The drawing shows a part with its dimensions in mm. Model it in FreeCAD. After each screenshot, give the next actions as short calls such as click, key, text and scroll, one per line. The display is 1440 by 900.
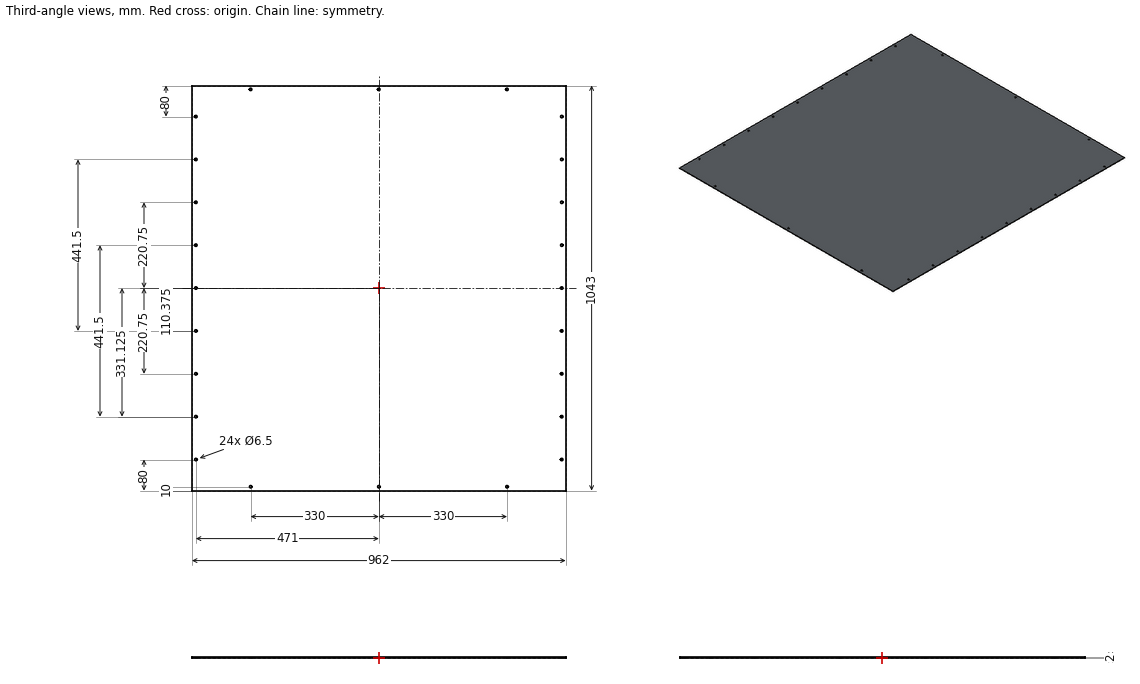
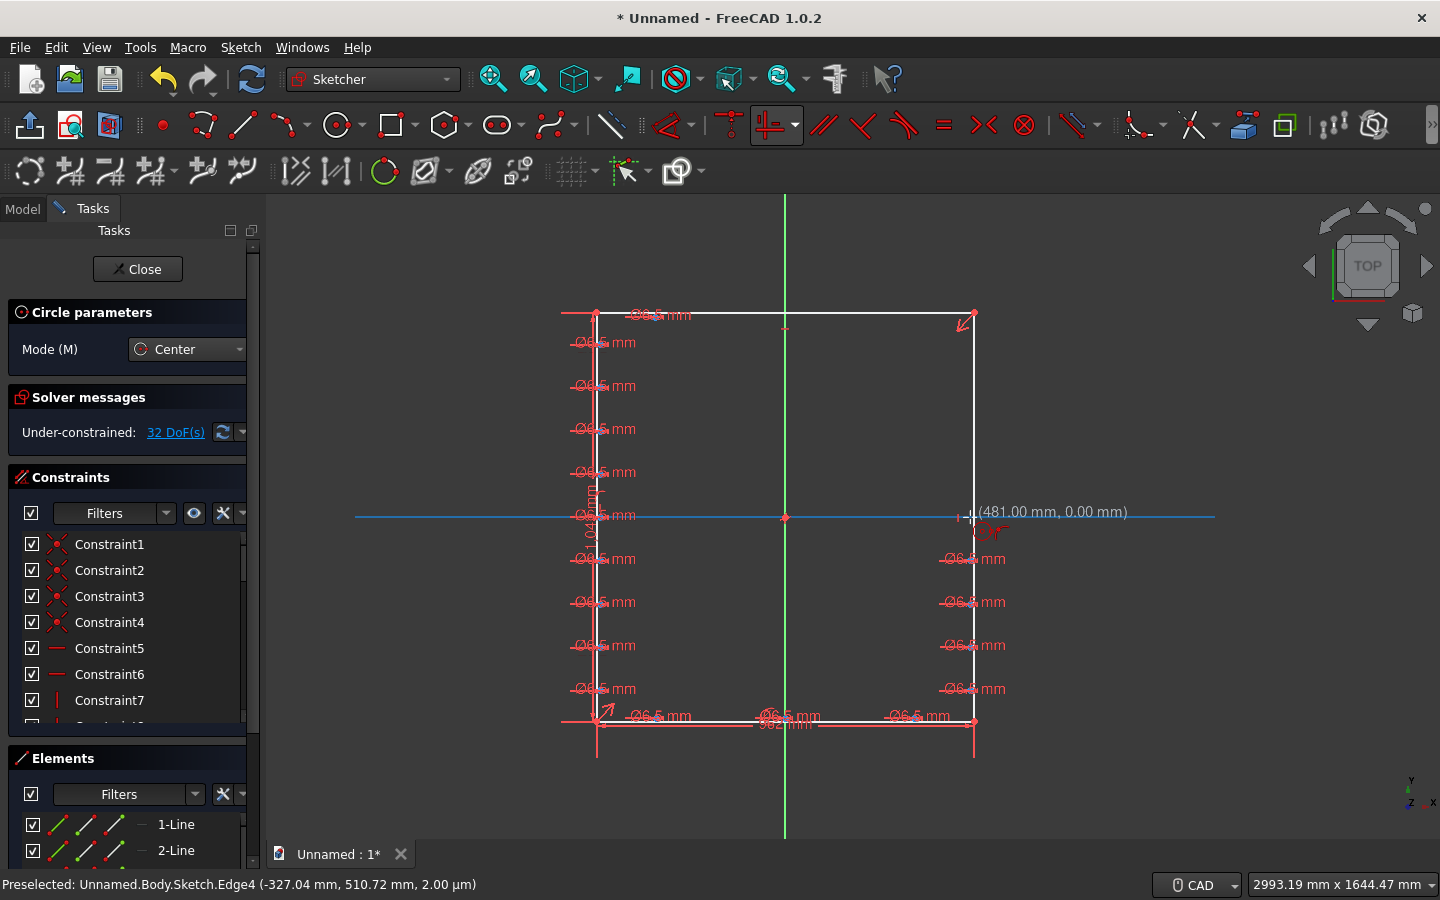
scroll(970, 517, up, 7)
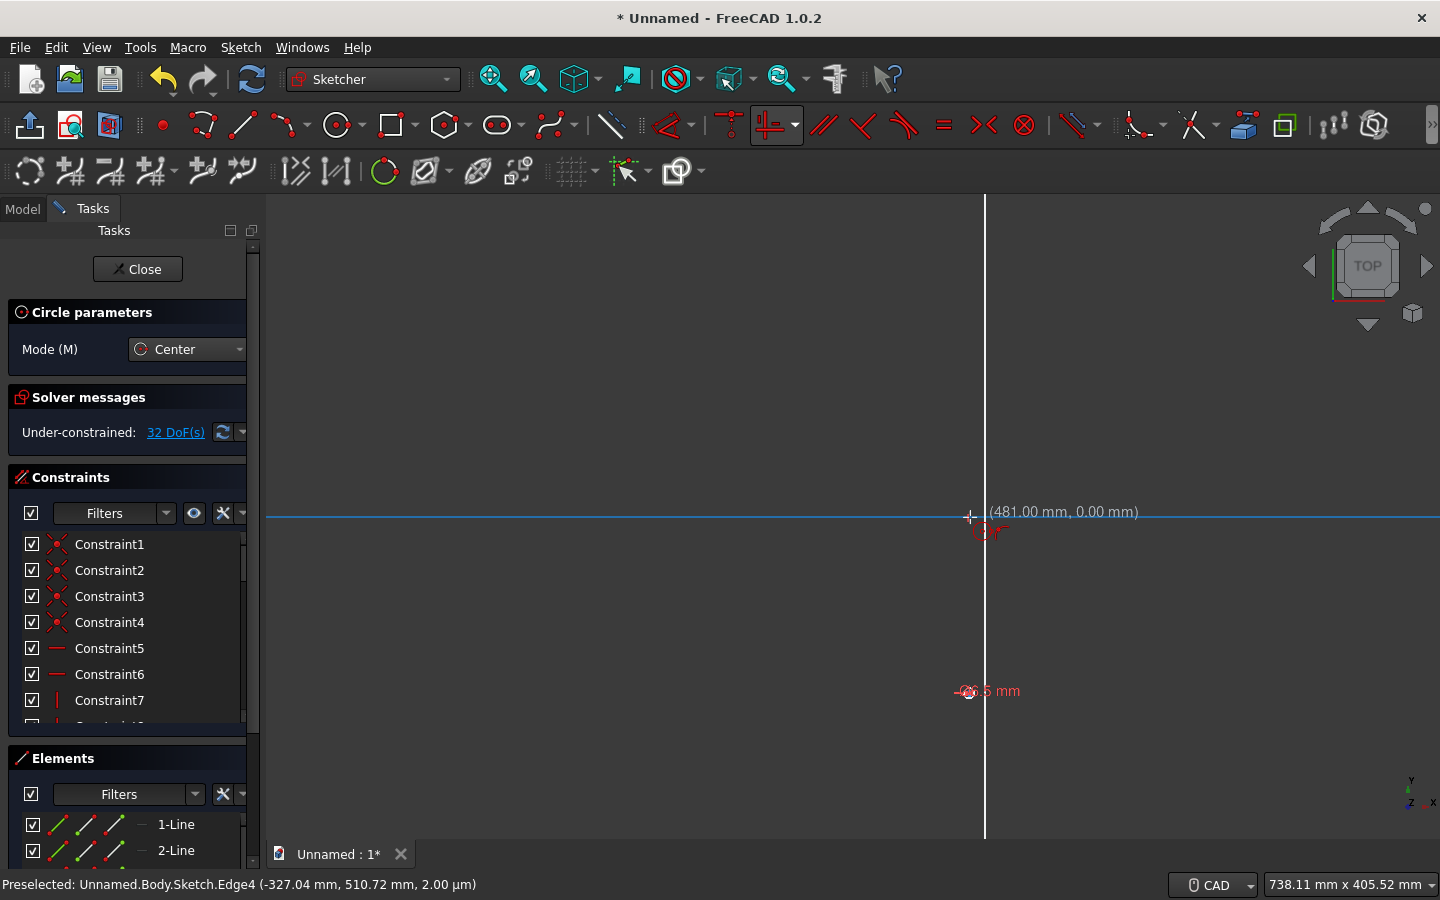
click(969, 517)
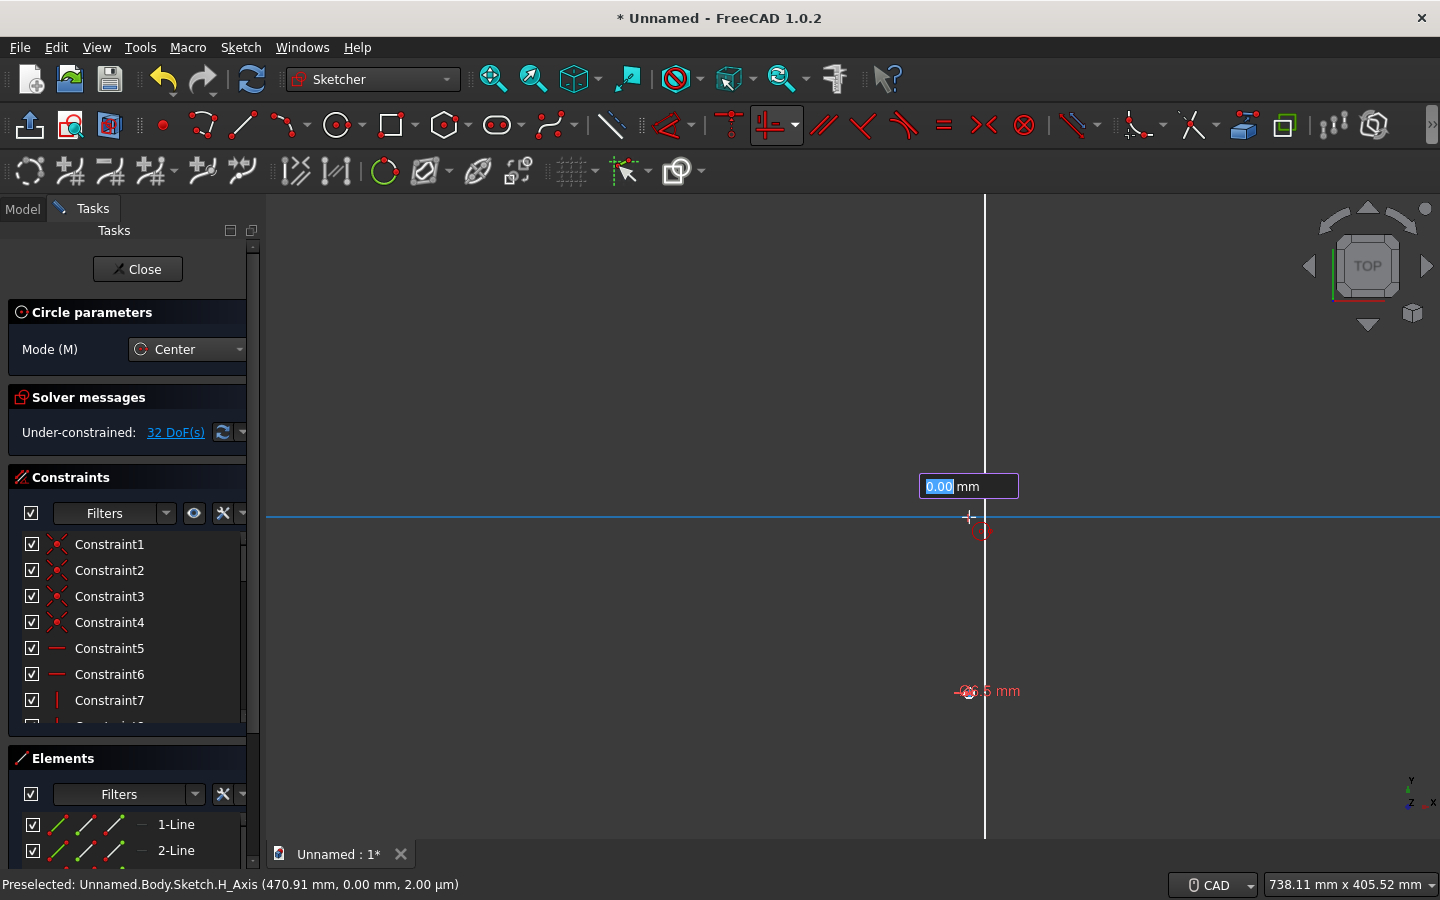
scroll(967, 522, up, 6)
move(967, 521)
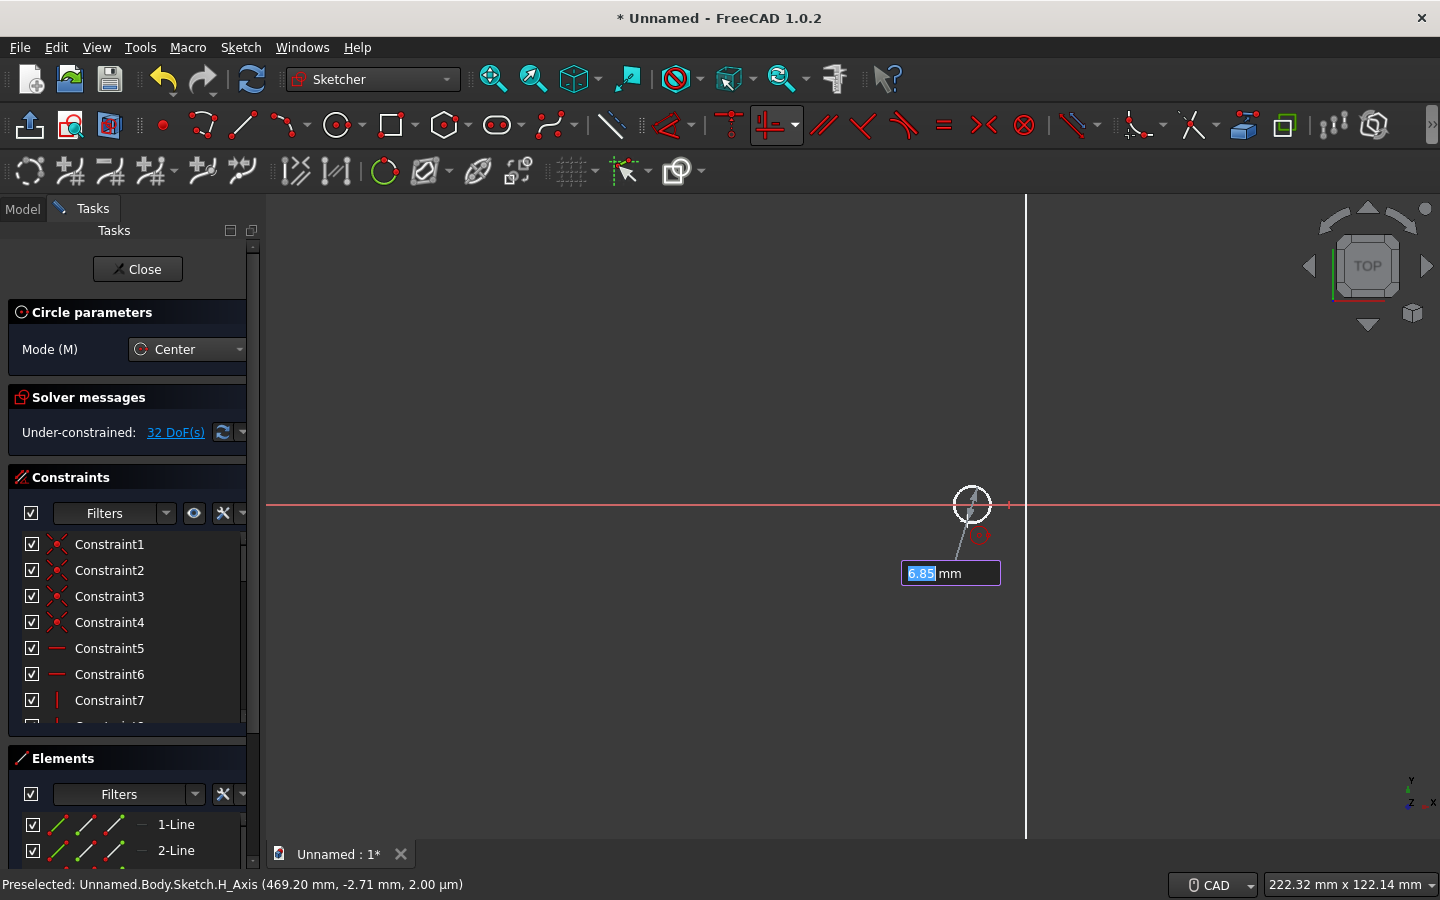
text(6.5)
key(Return)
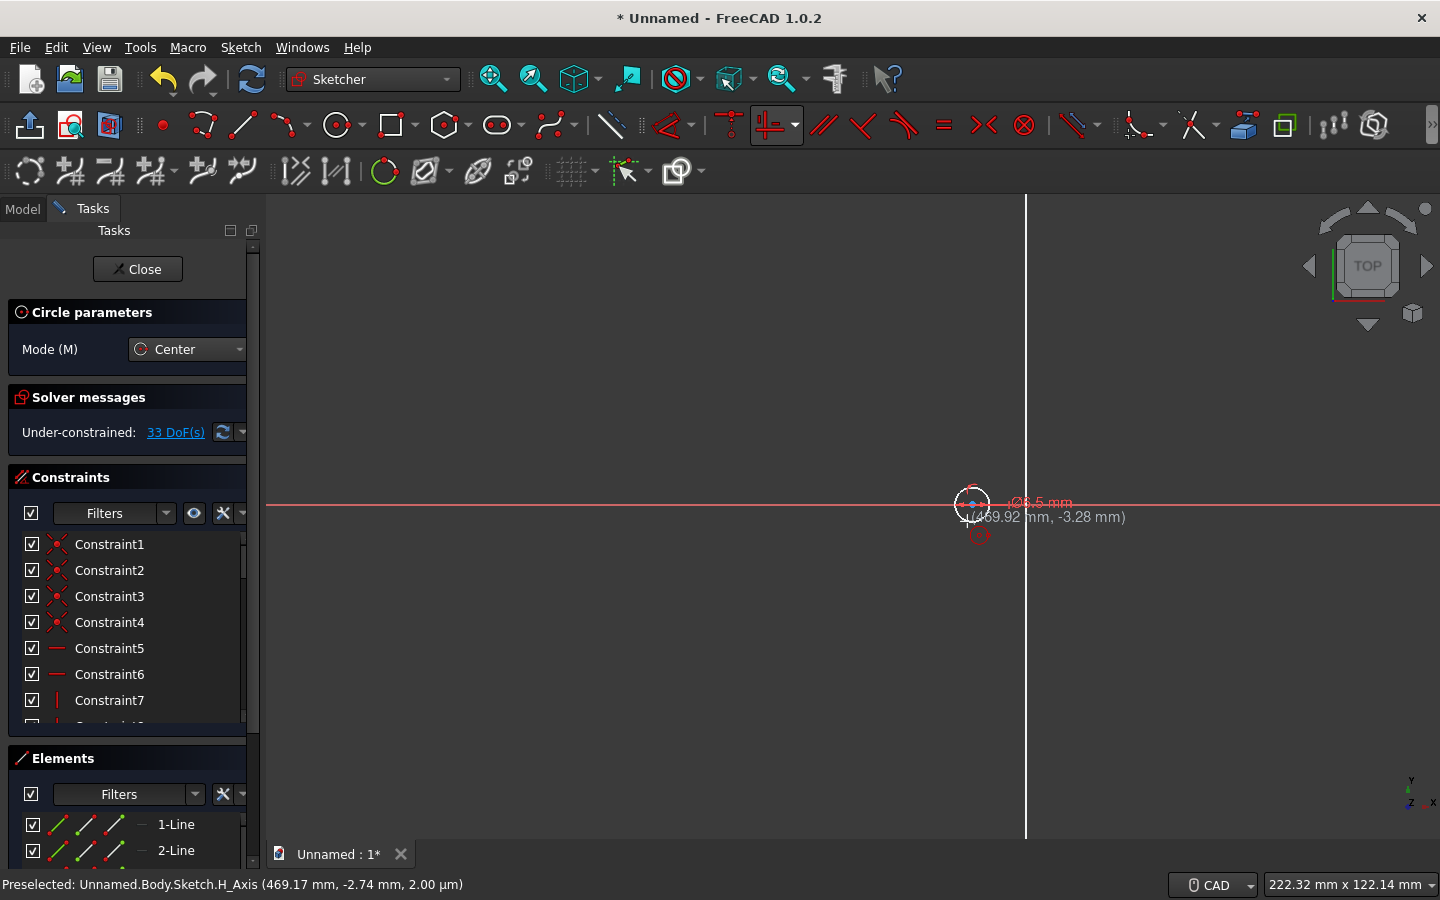
scroll(969, 517, down, 13)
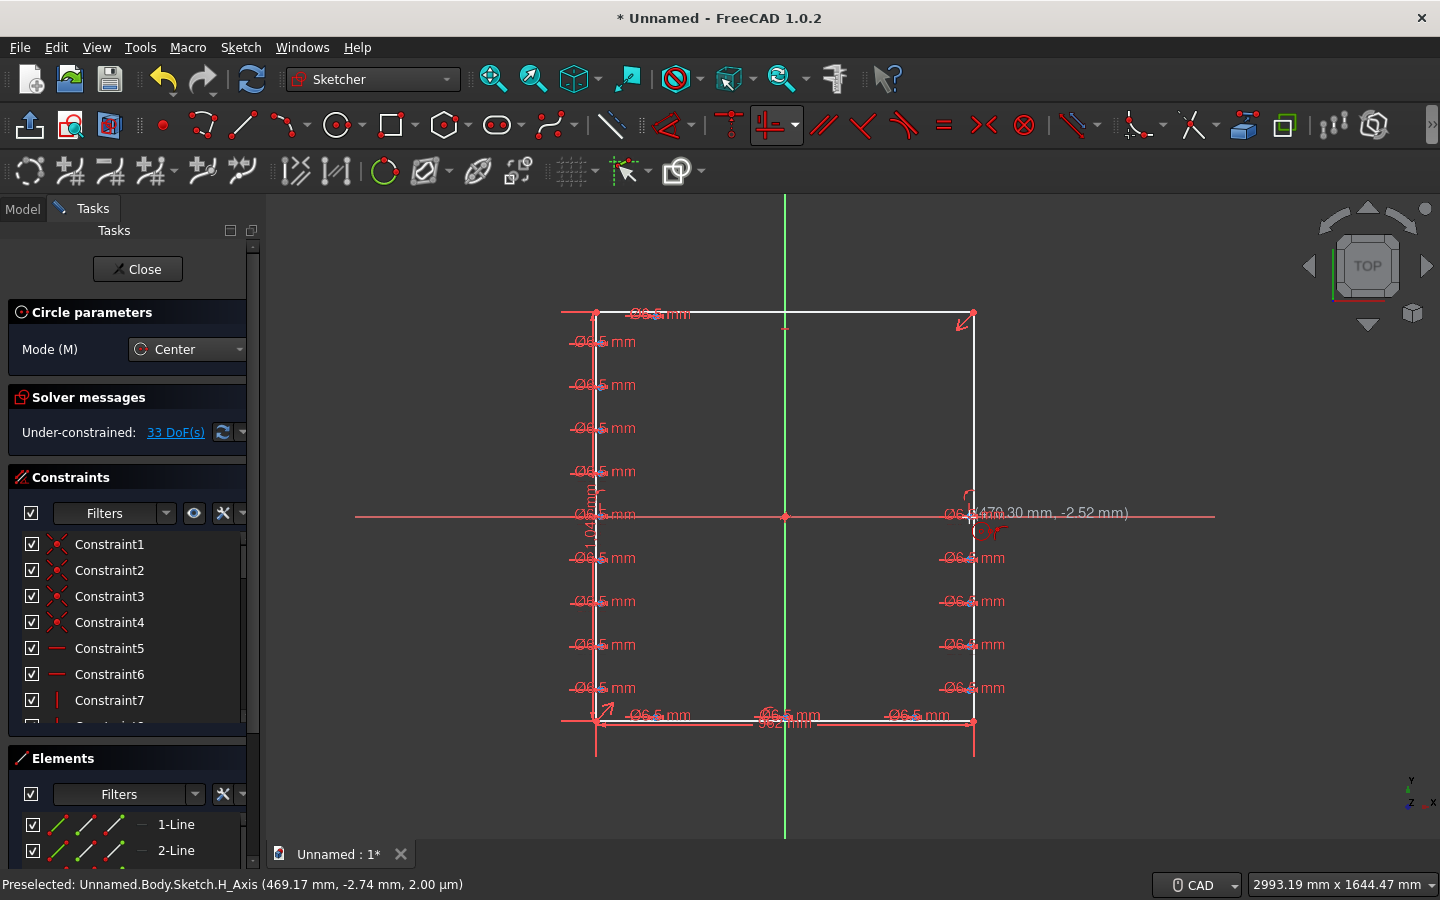
scroll(970, 473, up, 15)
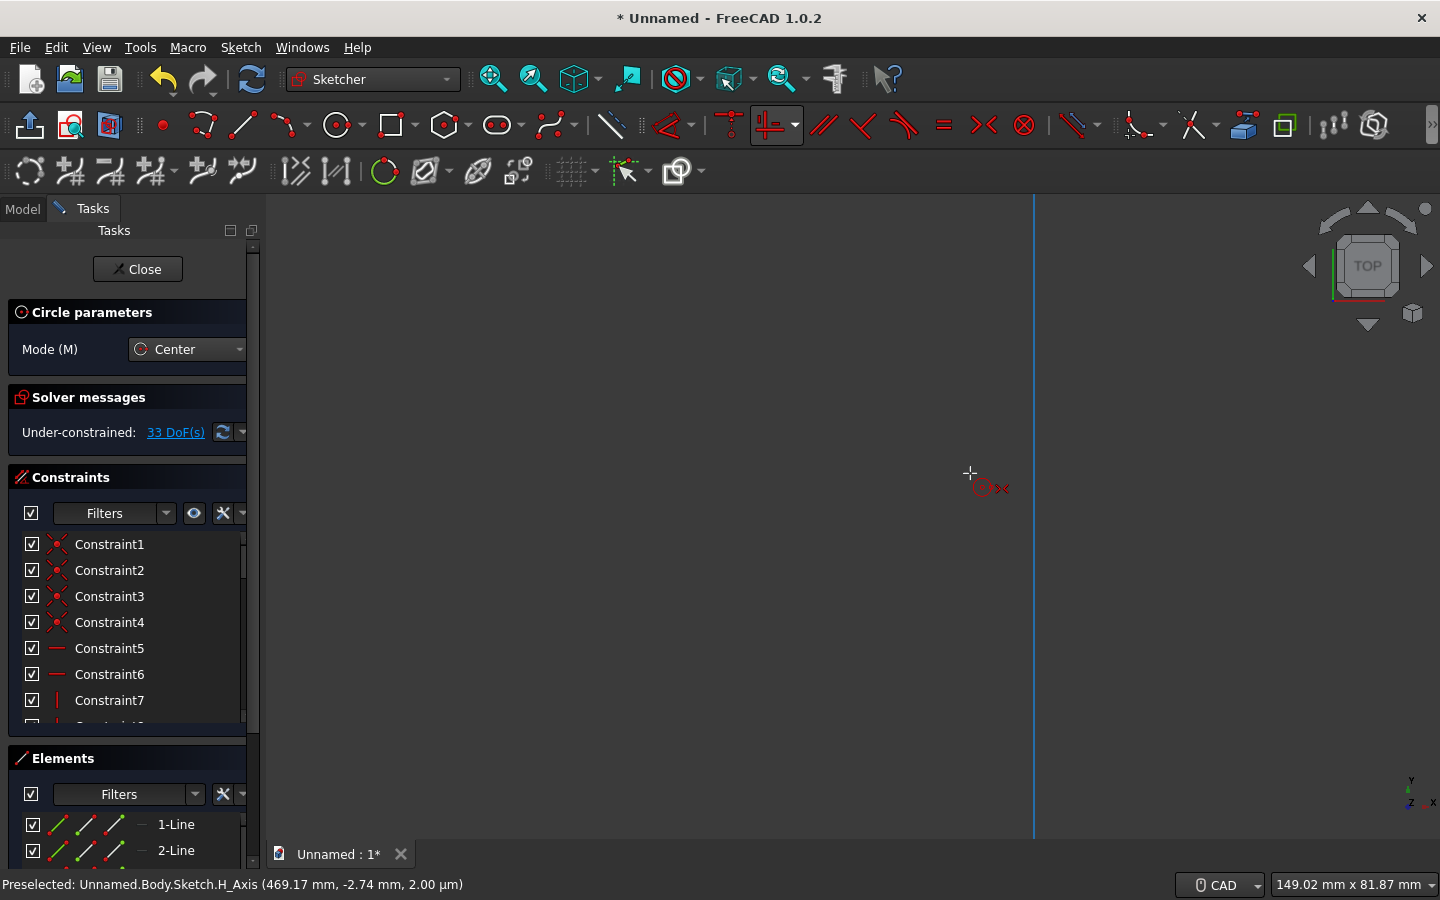
scroll(970, 473, down, 15)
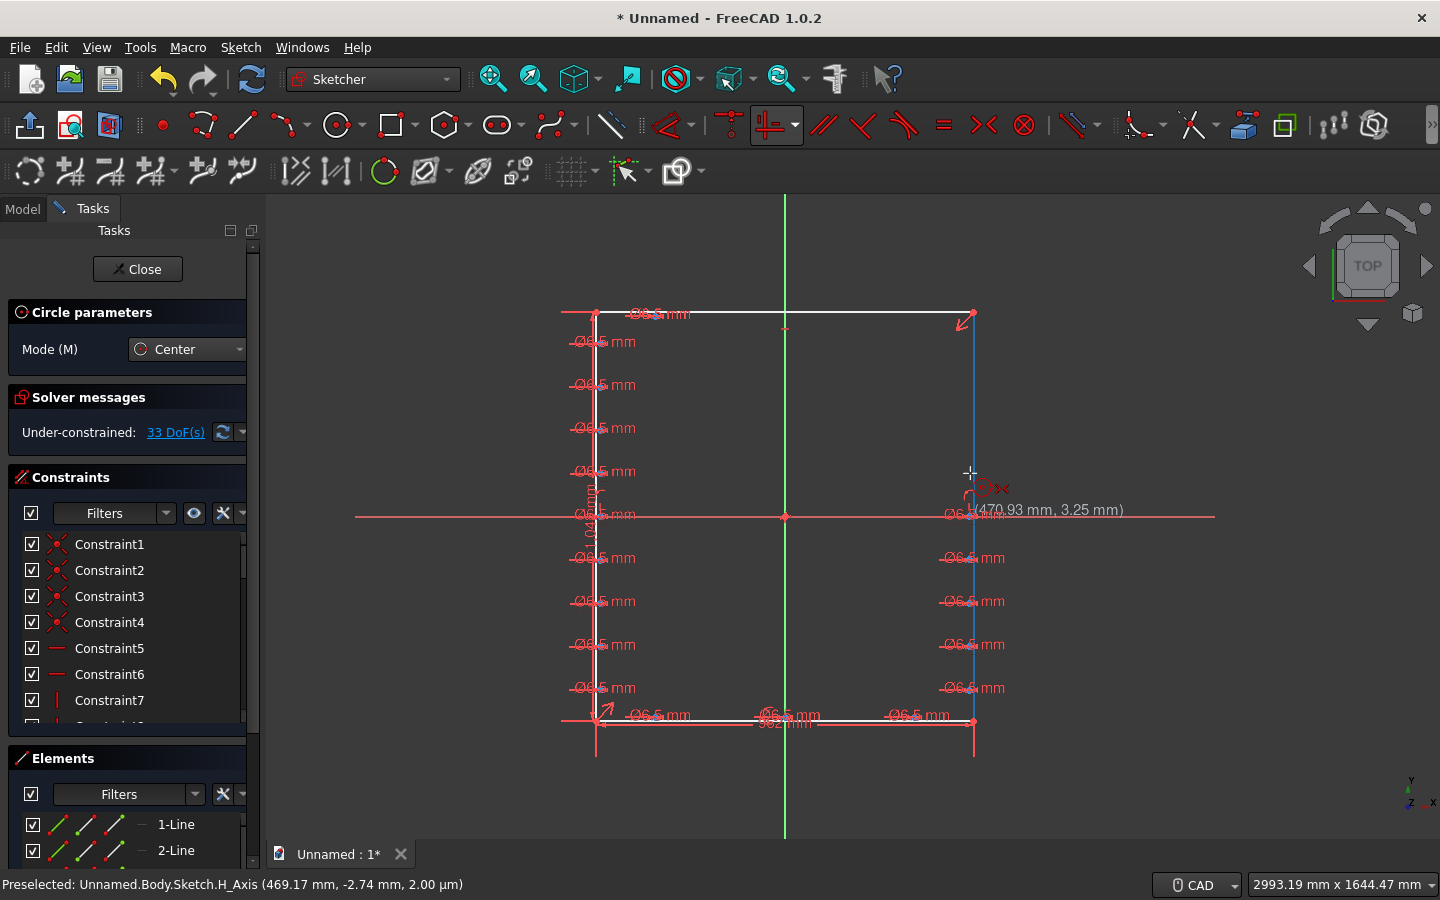
scroll(970, 473, up, 7)